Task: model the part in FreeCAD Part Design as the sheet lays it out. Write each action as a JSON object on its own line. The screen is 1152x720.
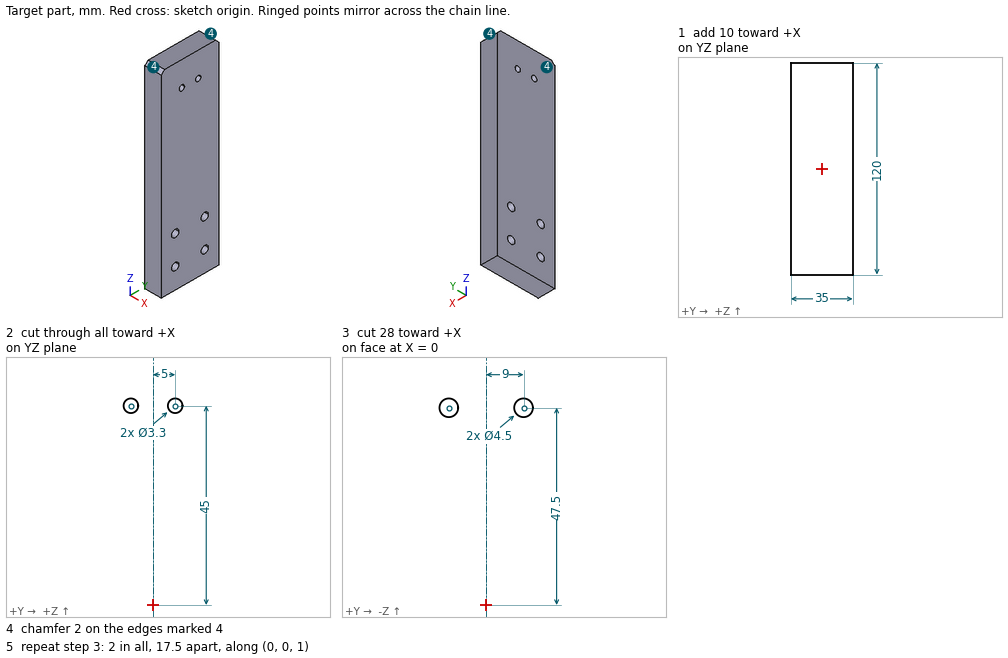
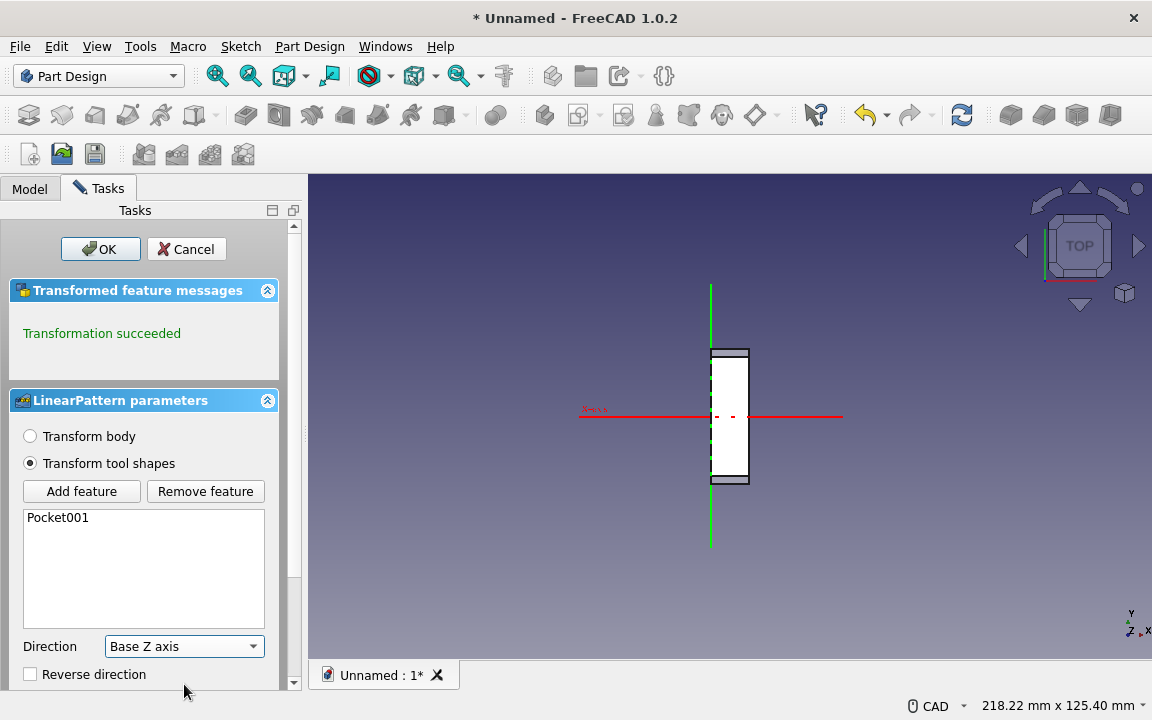
{"action": "scroll", "coordinate": [294, 455], "scroll_direction": "down", "scroll_amount": 2}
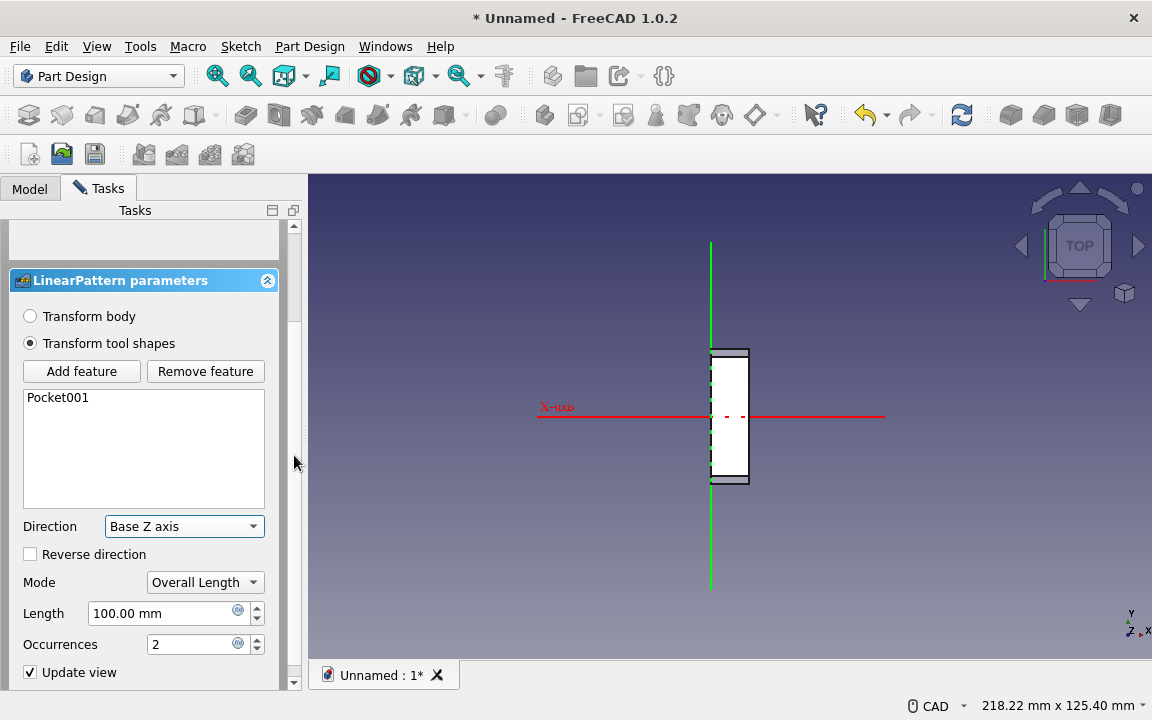
{"action": "left_click", "coordinate": [206, 582]}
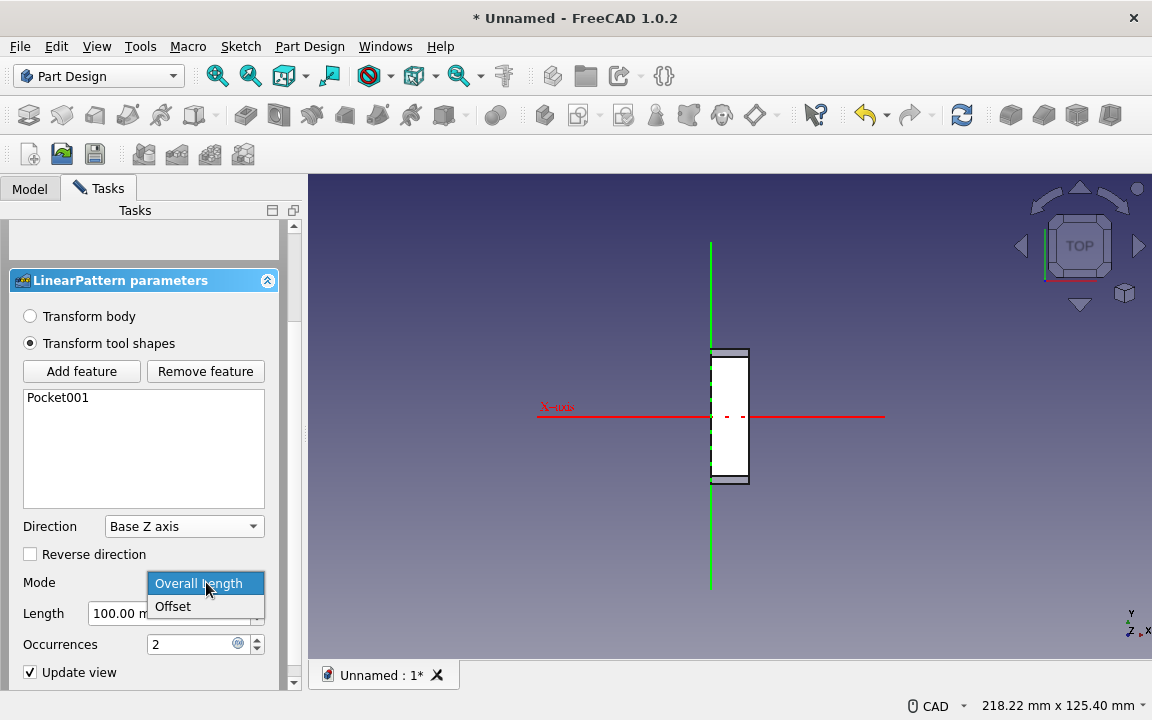
{"action": "left_click", "coordinate": [204, 606]}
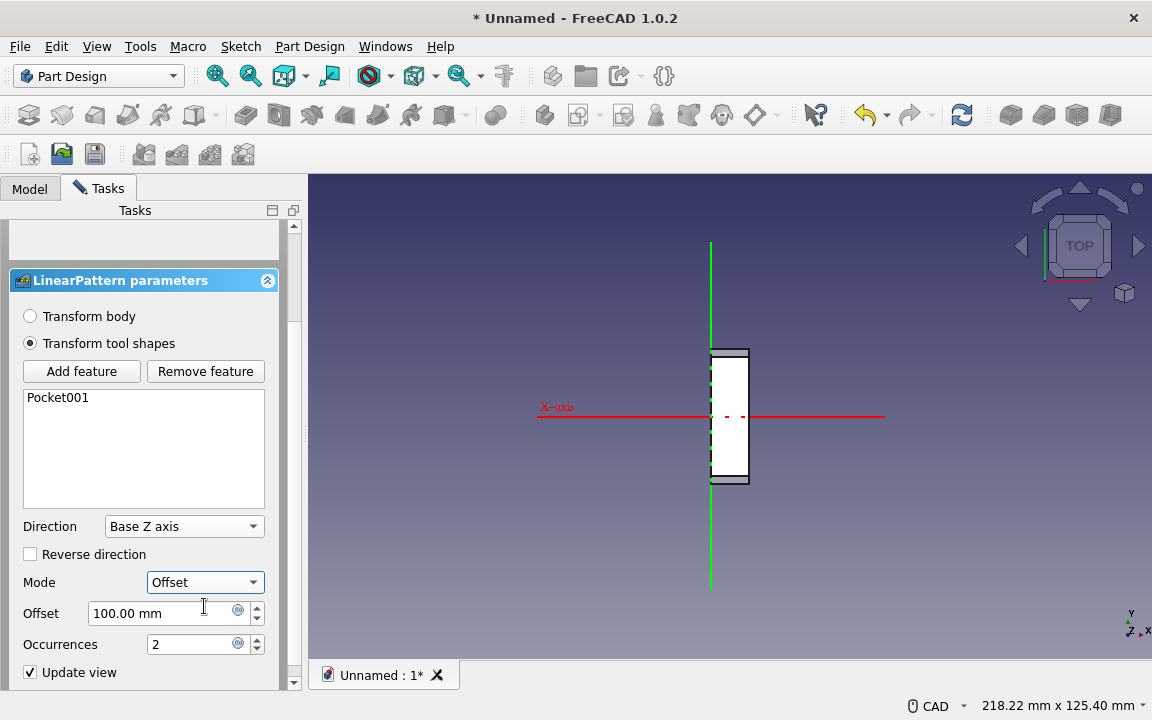
{"action": "triple_click", "coordinate": [170, 614]}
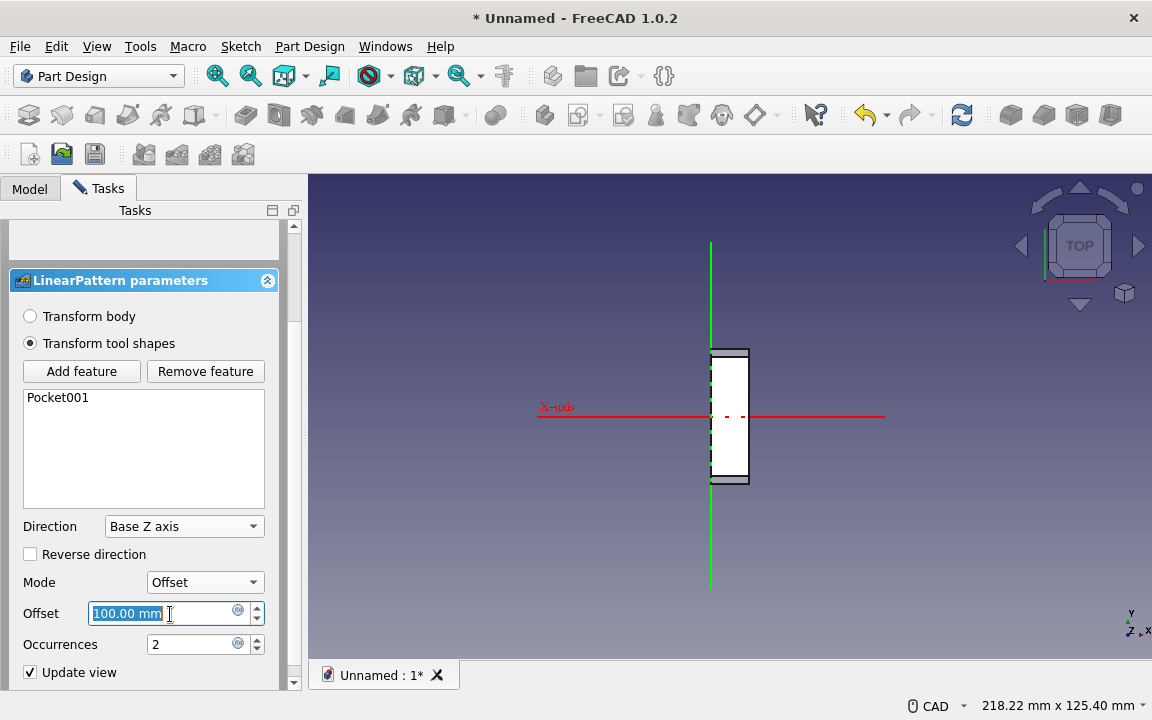
{"action": "type", "text": "17.5"}
{"action": "key", "text": "Tab"}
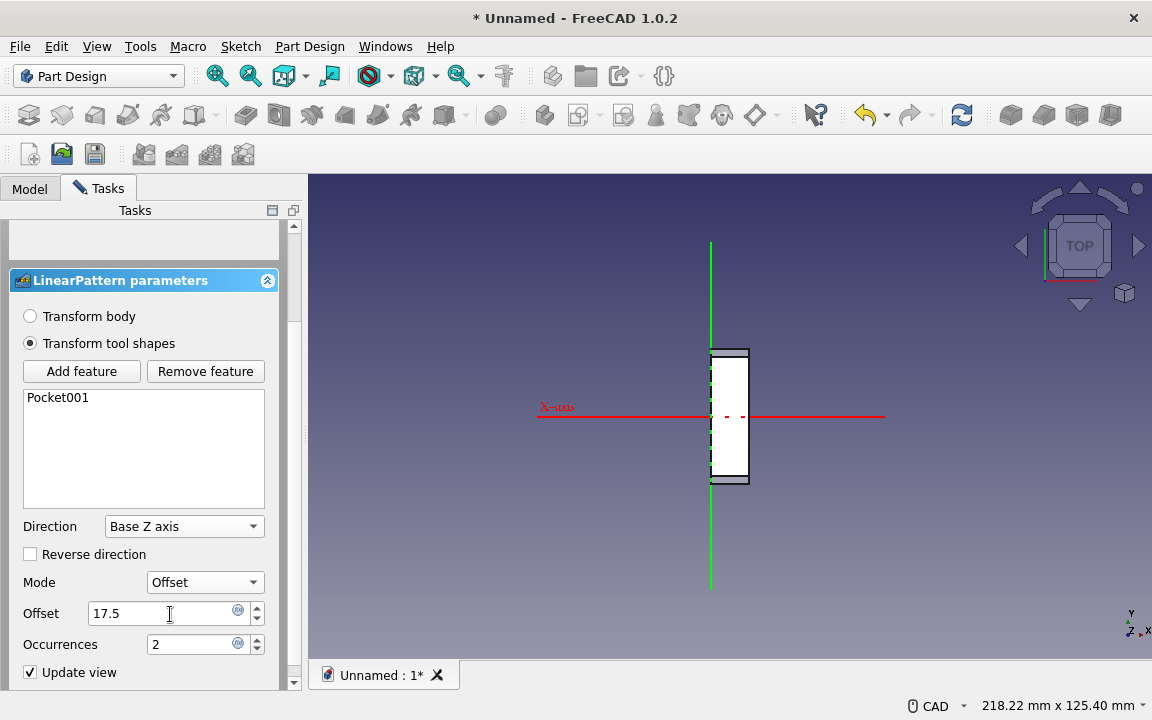
{"action": "triple_click", "coordinate": [199, 644]}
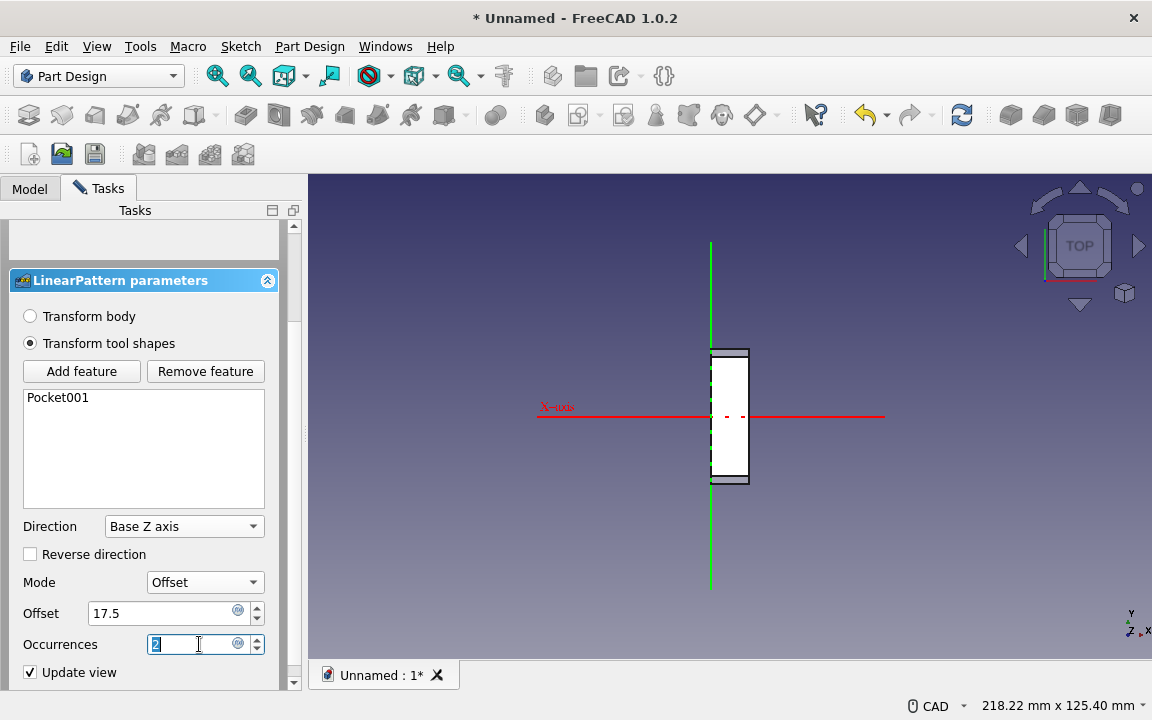
{"action": "type", "text": "2"}
{"action": "key", "text": "Tab"}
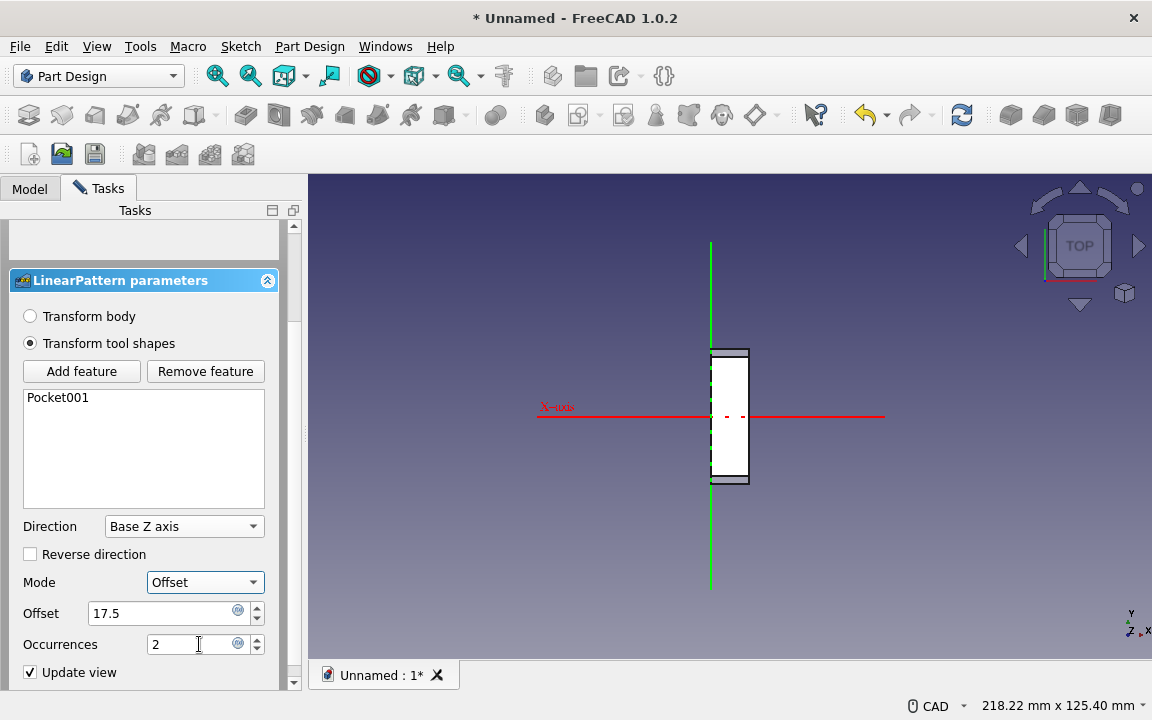
{"action": "scroll", "coordinate": [294, 455], "scroll_direction": "up", "scroll_amount": 3}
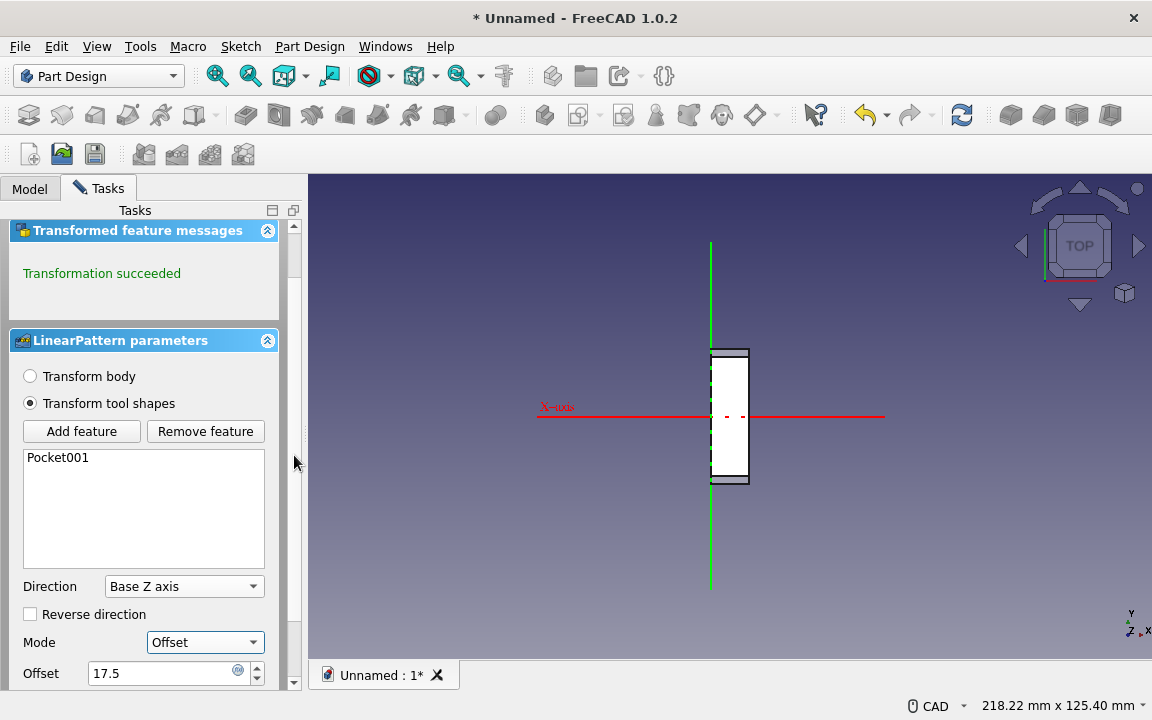
{"action": "left_click", "coordinate": [101, 249]}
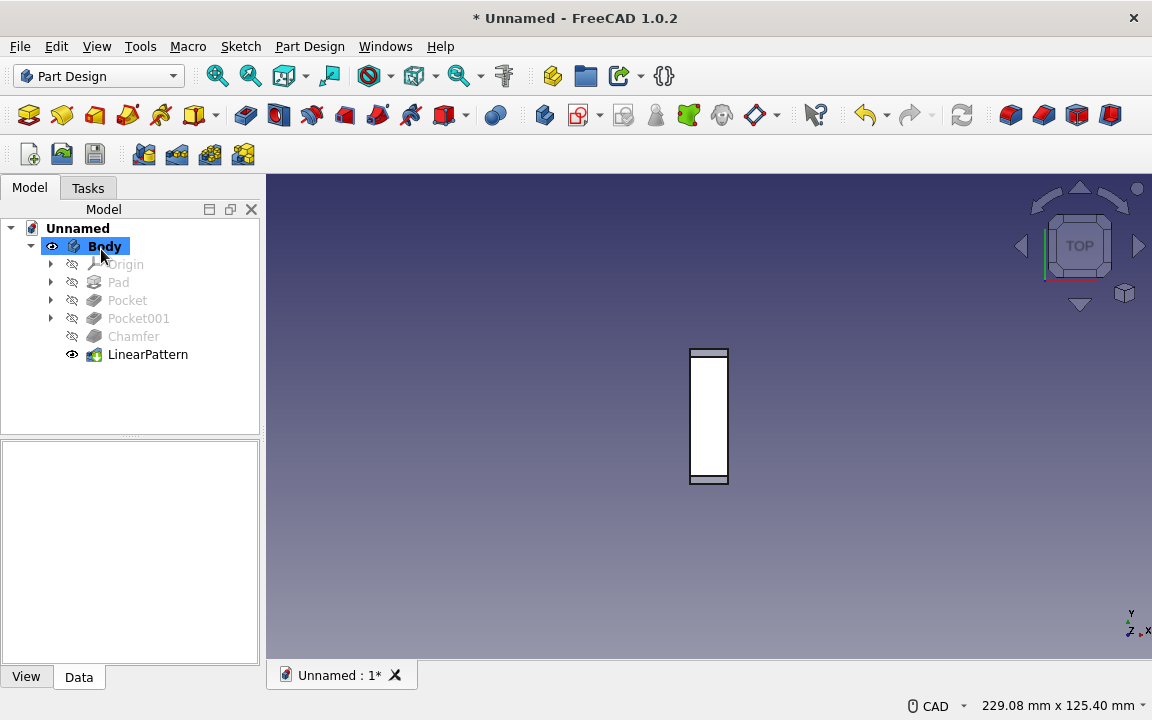
{"action": "key", "text": "0"}